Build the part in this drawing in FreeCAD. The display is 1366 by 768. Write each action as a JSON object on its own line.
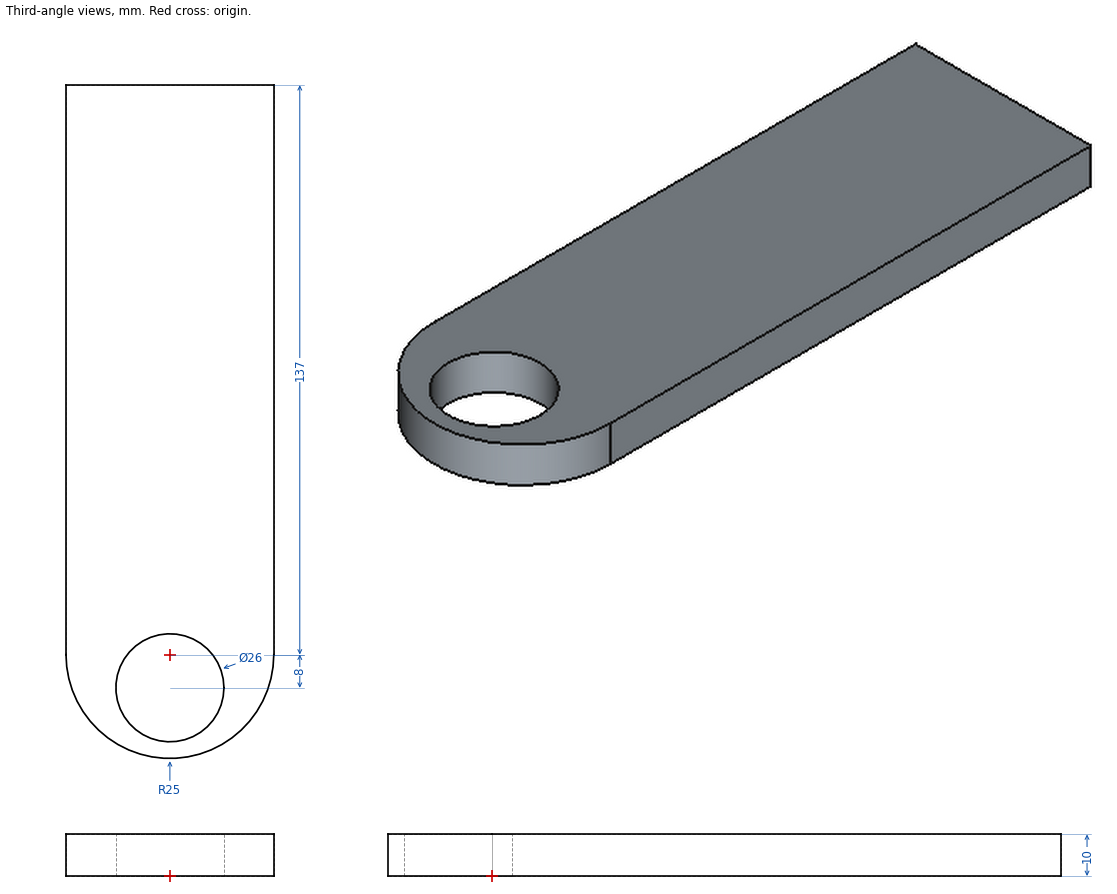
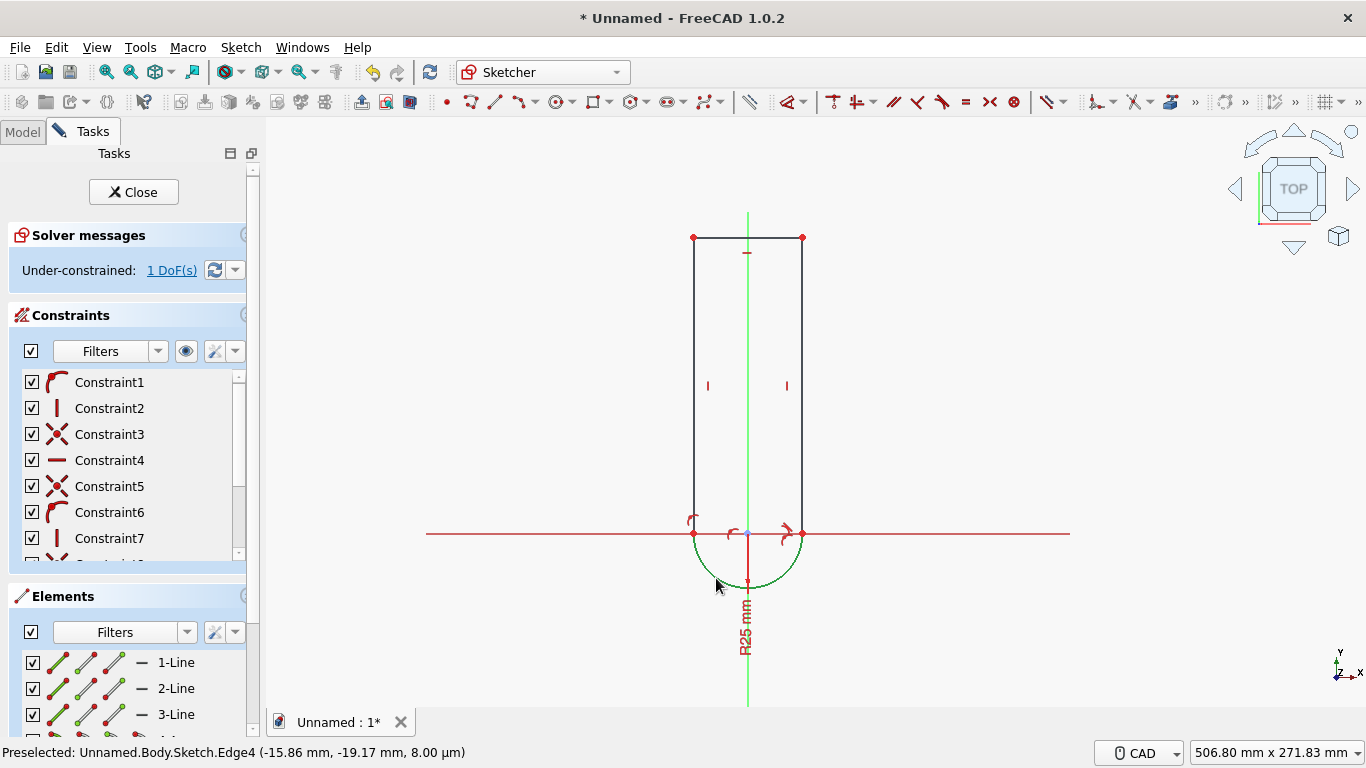
{"action": "left_click", "coordinate": [802, 445]}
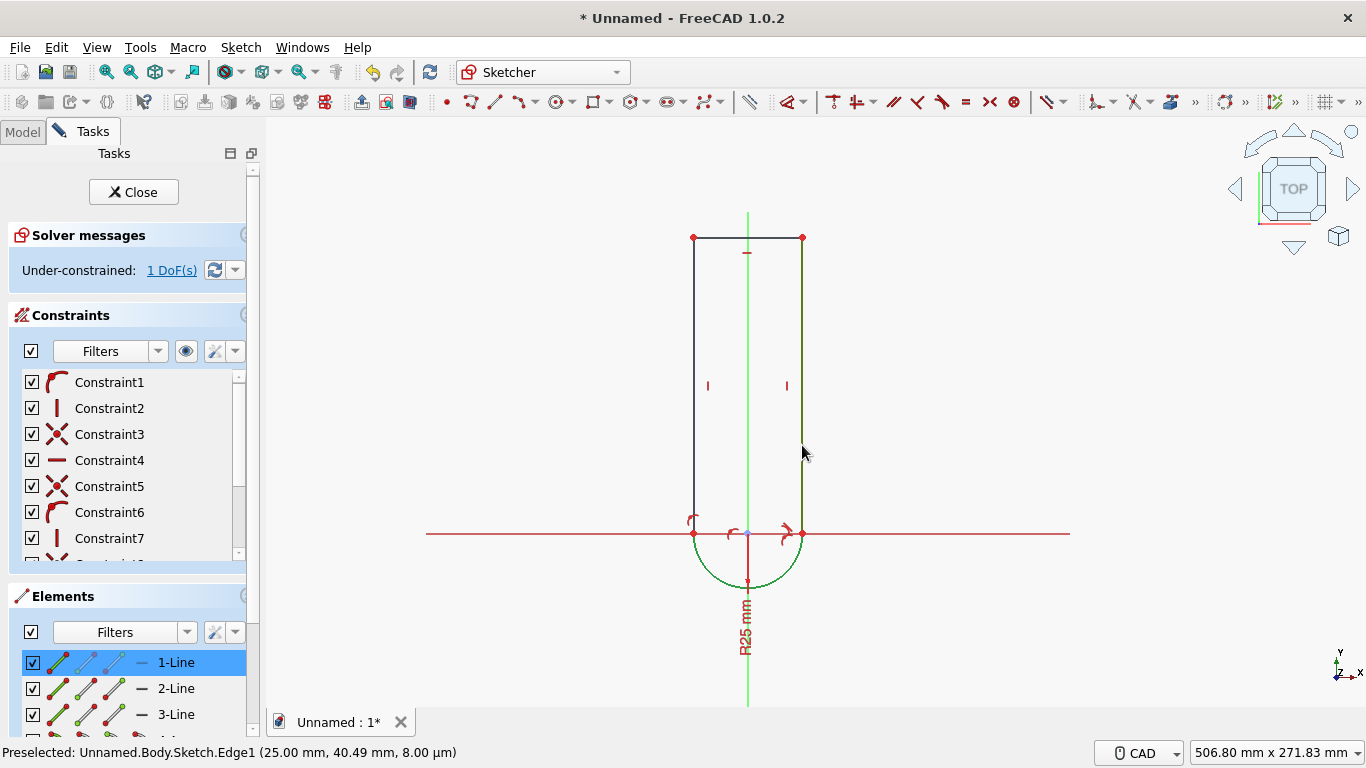
{"action": "key", "text": "i"}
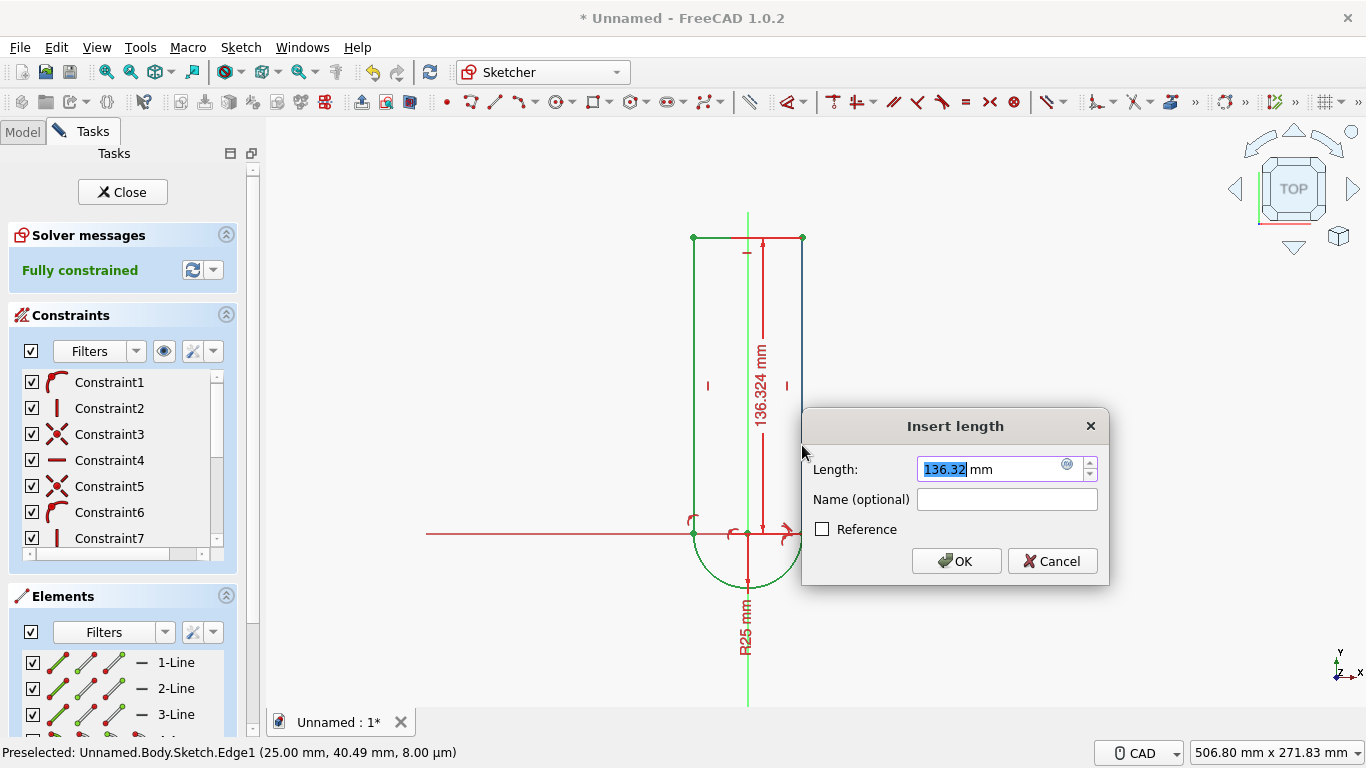
{"action": "type", "text": "137"}
{"action": "key", "text": "Return"}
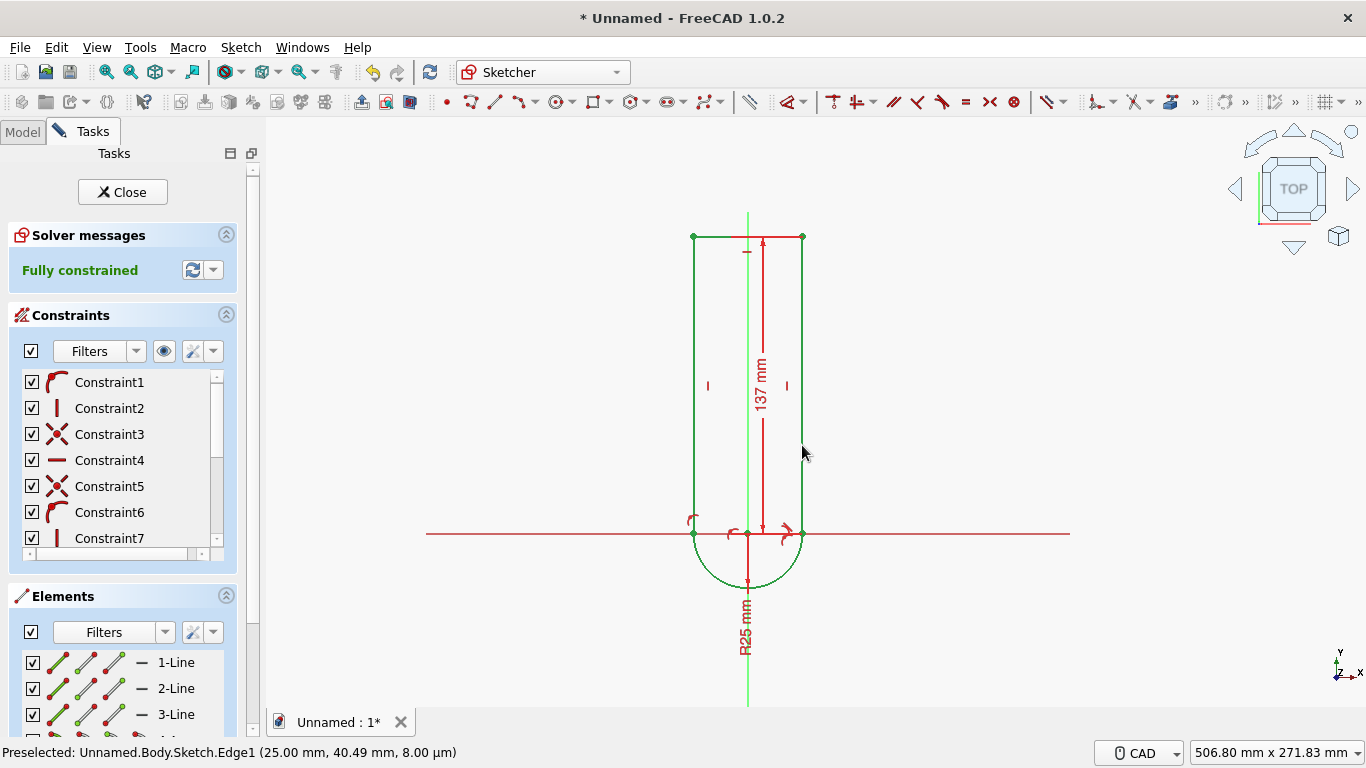
{"action": "left_click", "coordinate": [123, 192]}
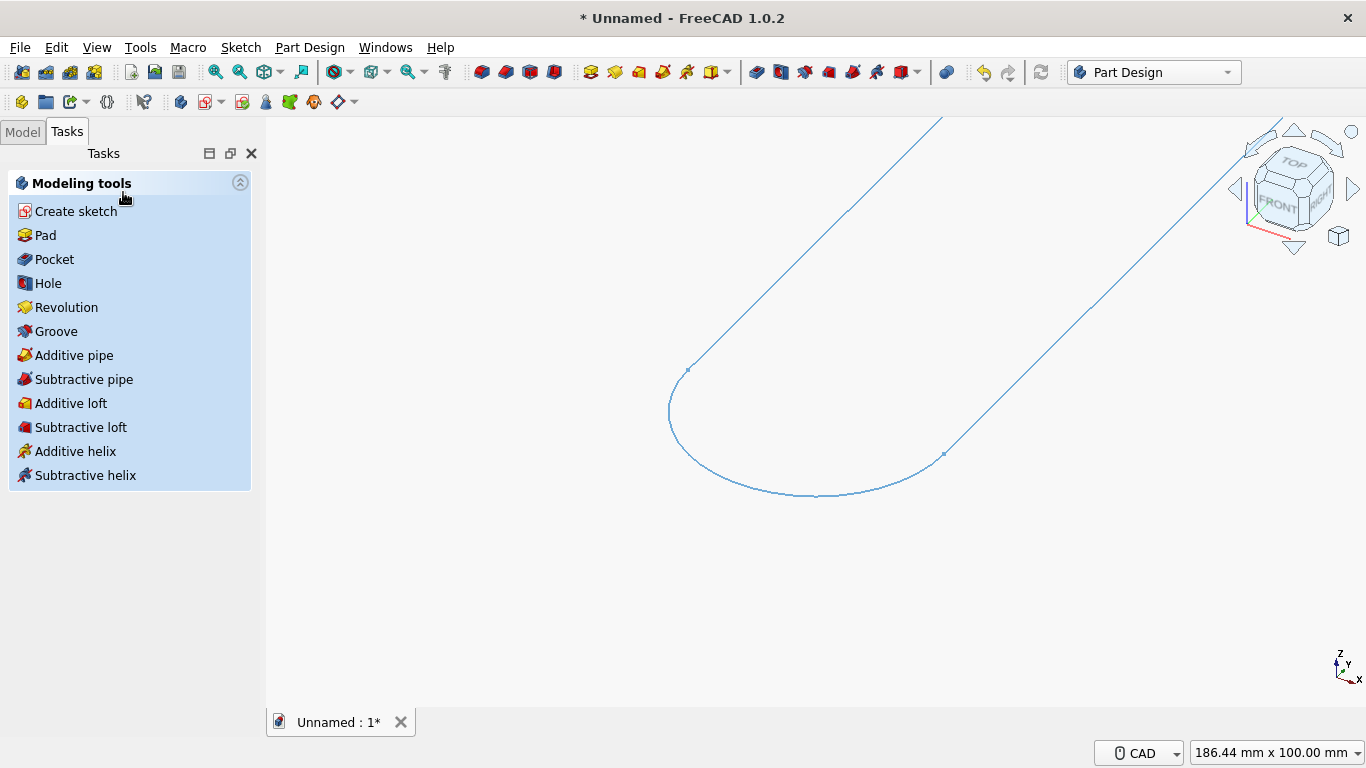
{"action": "left_click", "coordinate": [592, 72]}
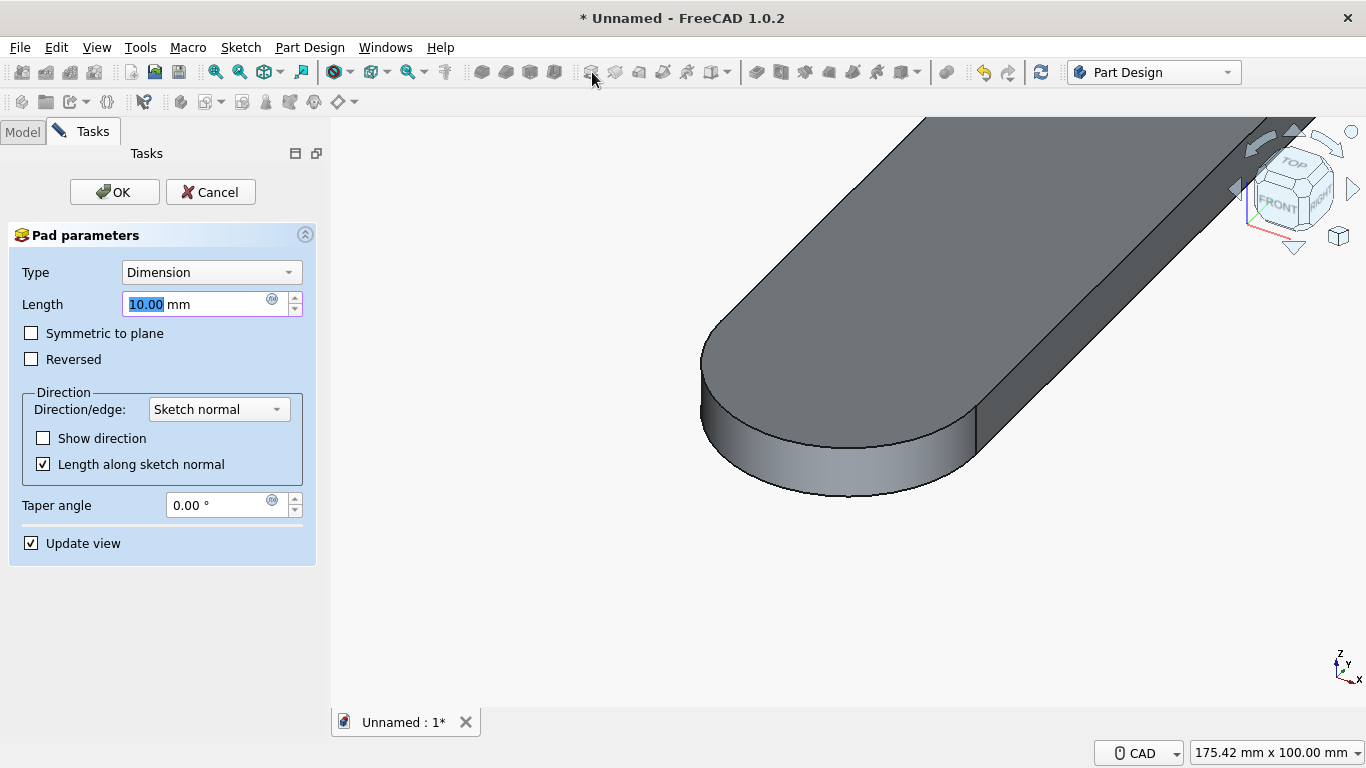
{"action": "type", "text": "10"}
{"action": "key", "text": "Tab"}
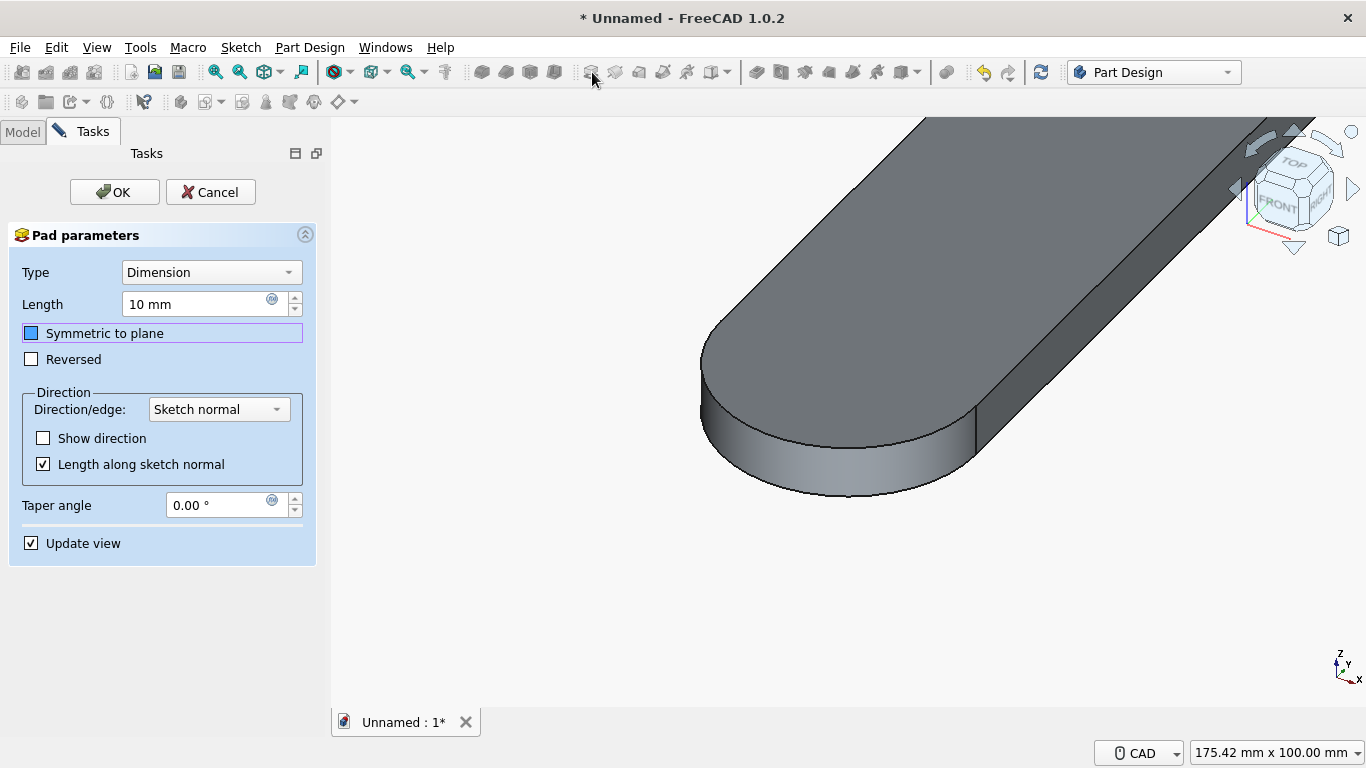
{"action": "left_click", "coordinate": [115, 192]}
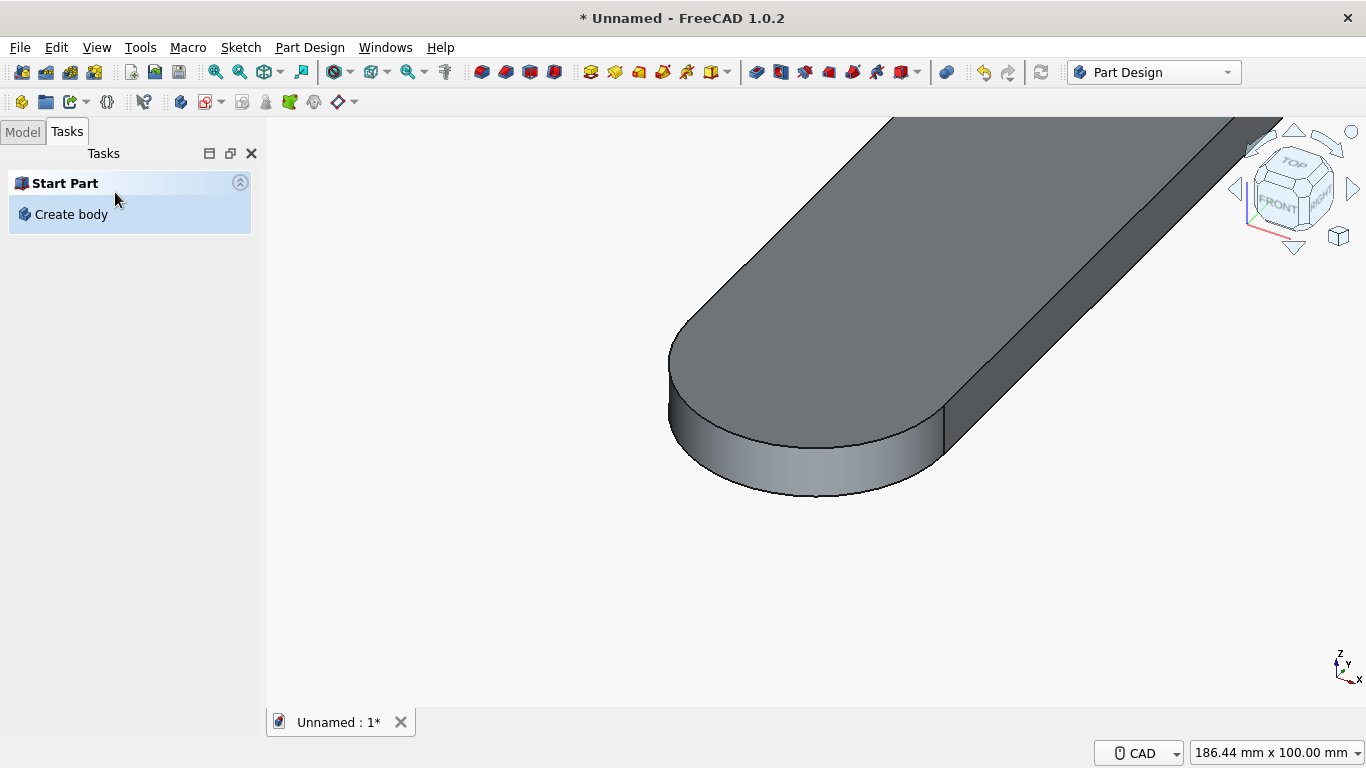
{"action": "left_click", "coordinate": [216, 72]}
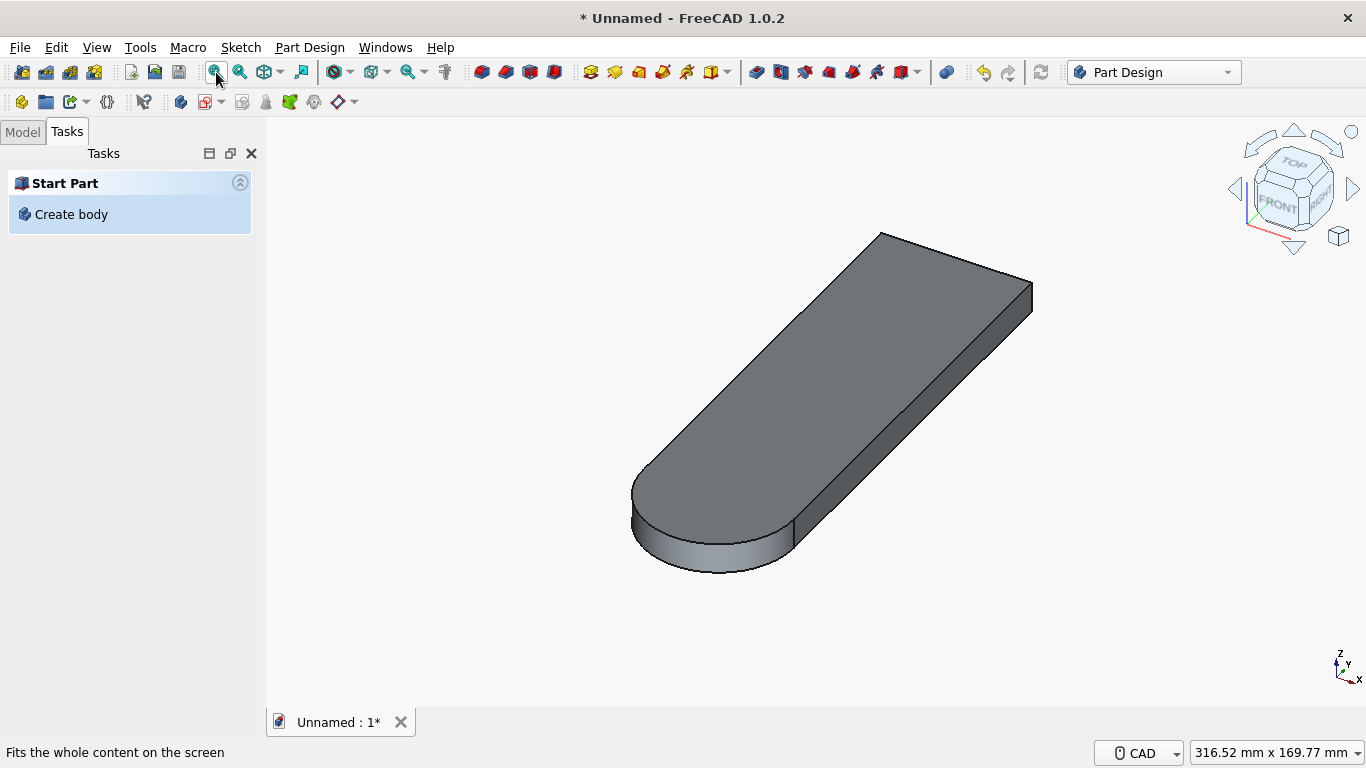
{"action": "left_click", "coordinate": [896, 317]}